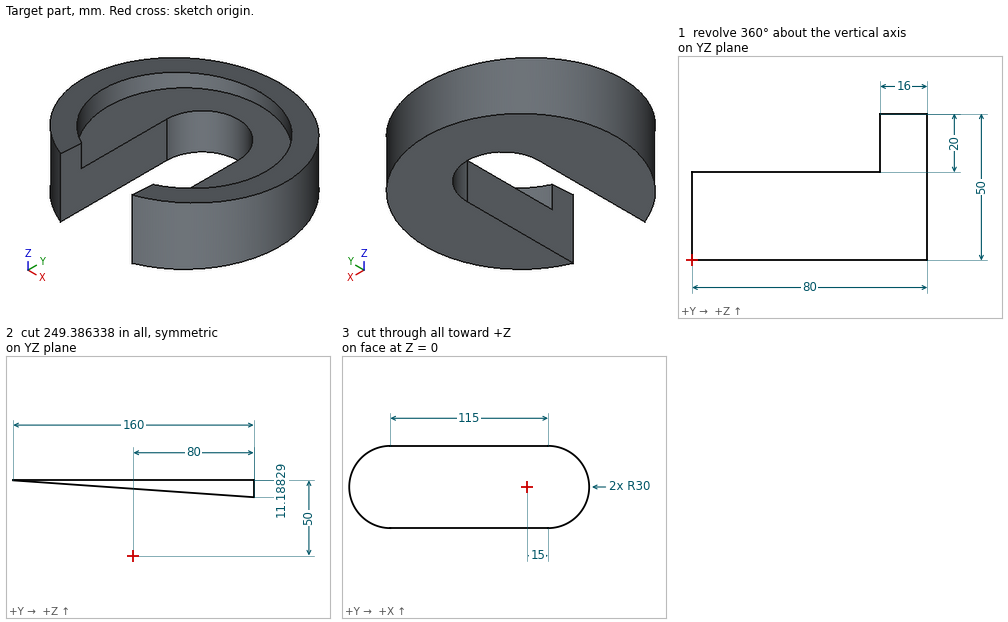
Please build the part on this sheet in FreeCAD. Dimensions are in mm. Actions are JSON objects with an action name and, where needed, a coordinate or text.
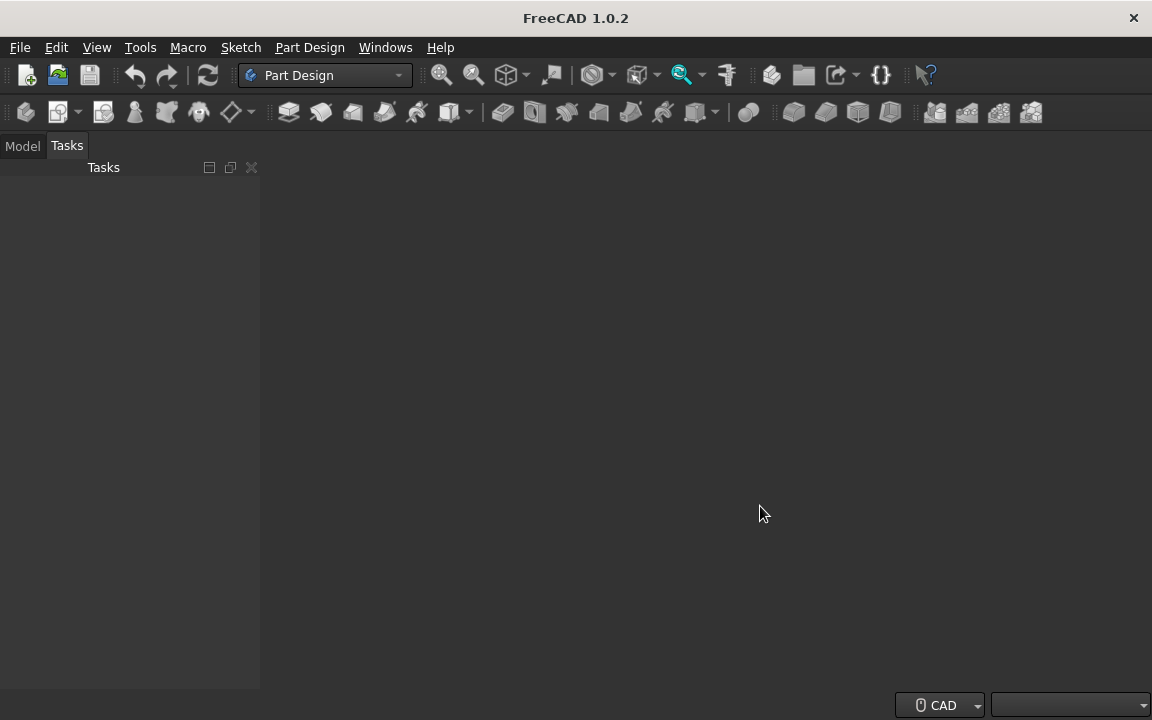
{"action": "left_click", "coordinate": [26, 76]}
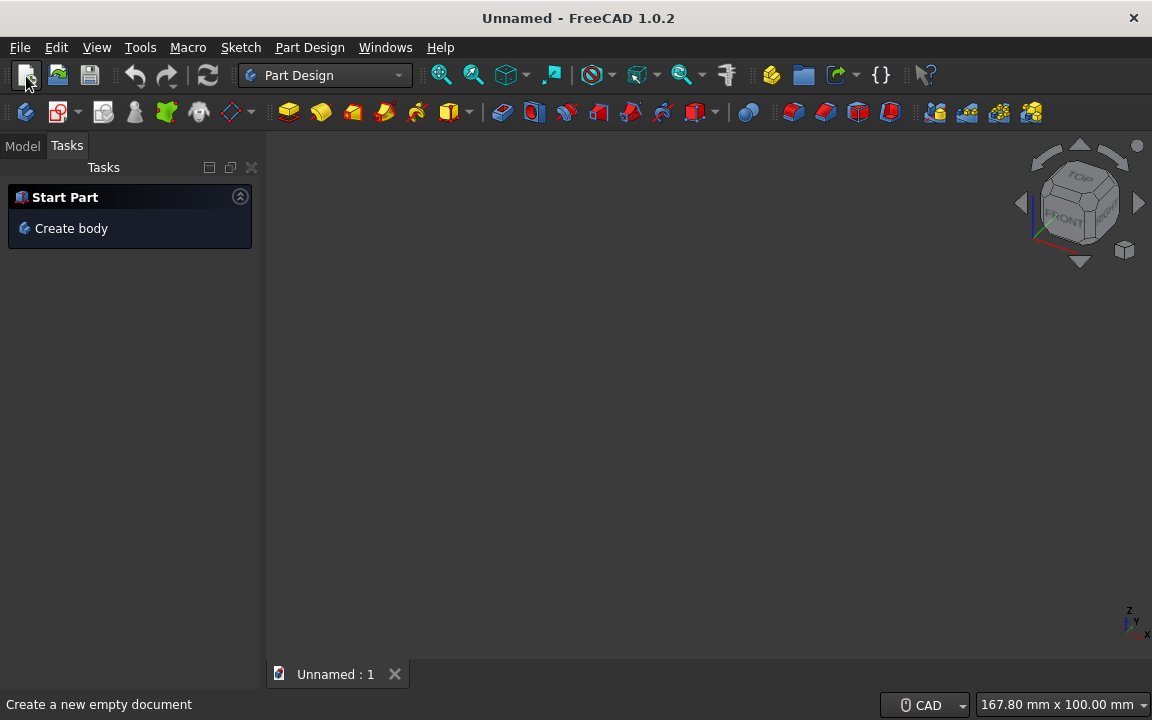
{"action": "left_click", "coordinate": [58, 112]}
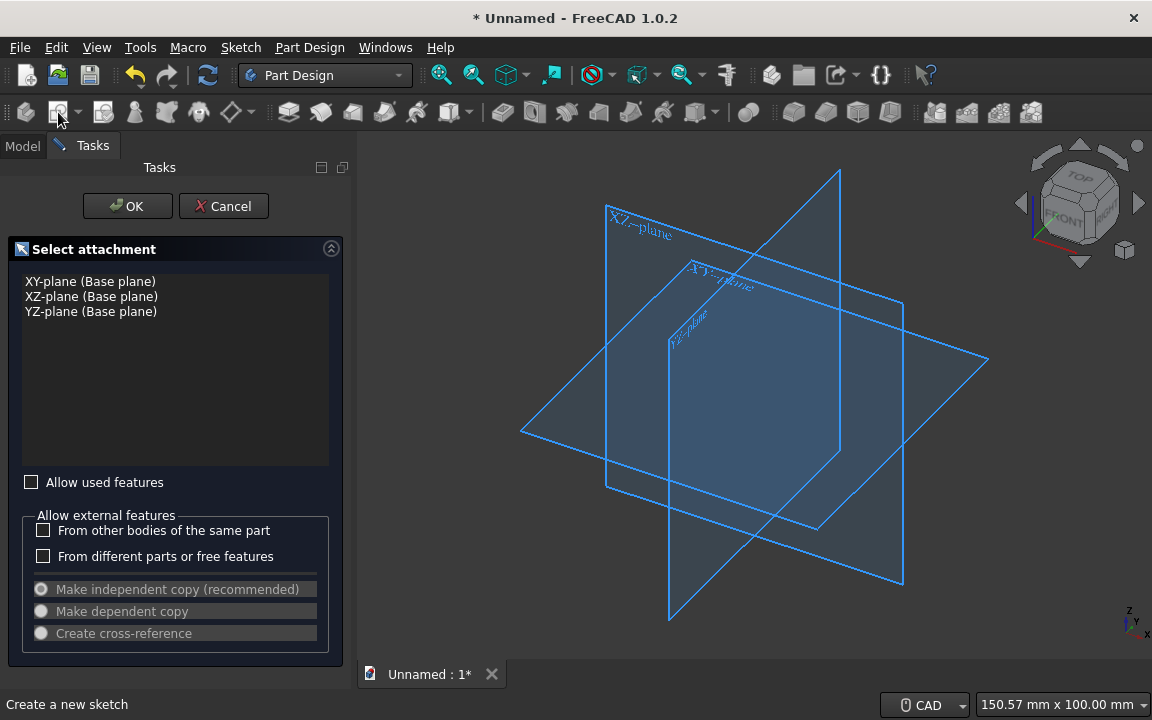
{"action": "left_click", "coordinate": [82, 312]}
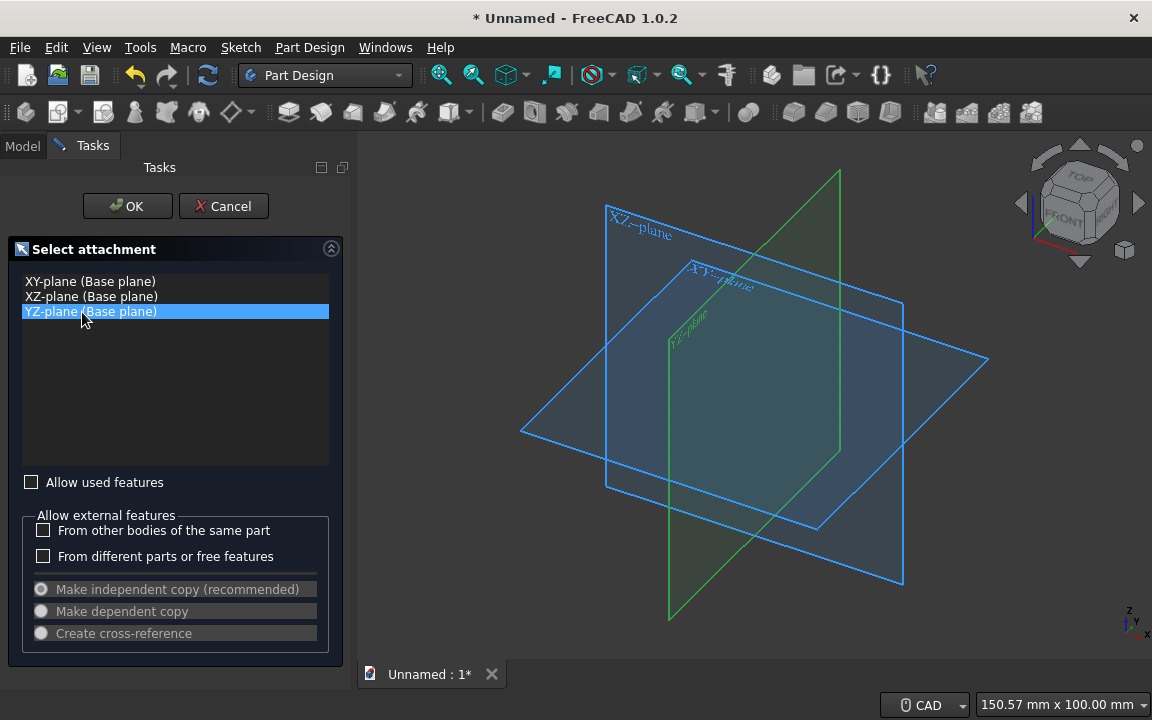
{"action": "left_click", "coordinate": [128, 206]}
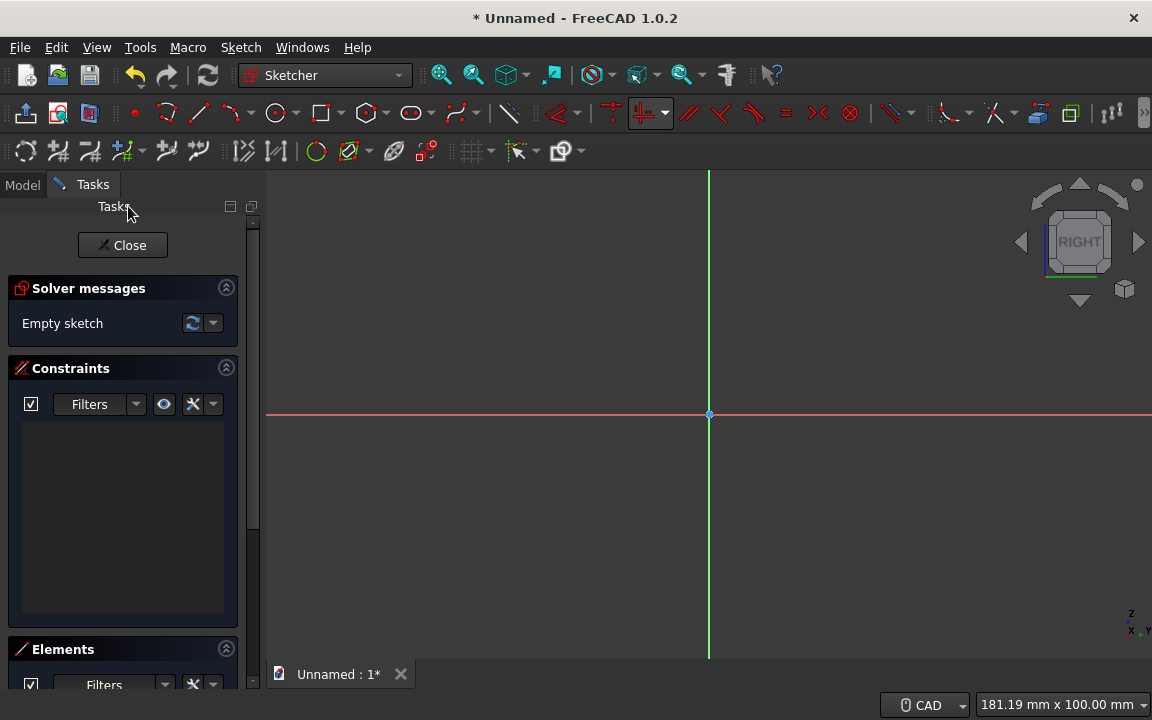
{"action": "scroll", "coordinate": [294, 631], "scroll_direction": "down", "scroll_amount": 1}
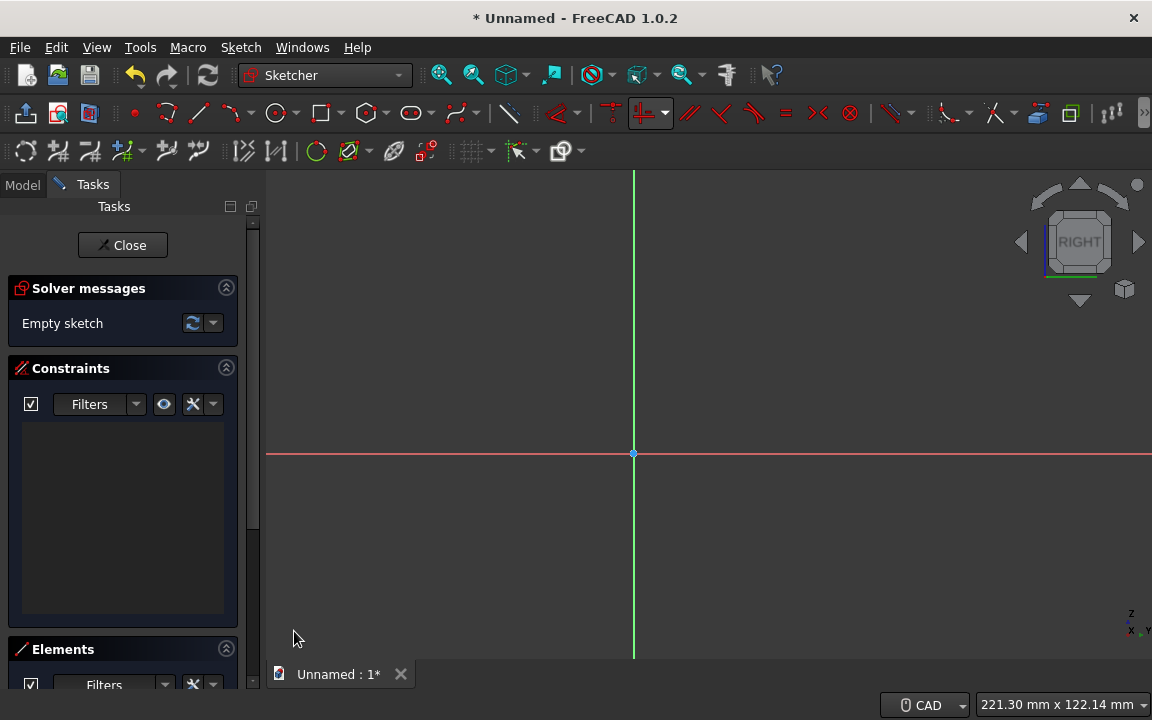
{"action": "scroll", "coordinate": [987, 230], "scroll_direction": "up", "scroll_amount": 2}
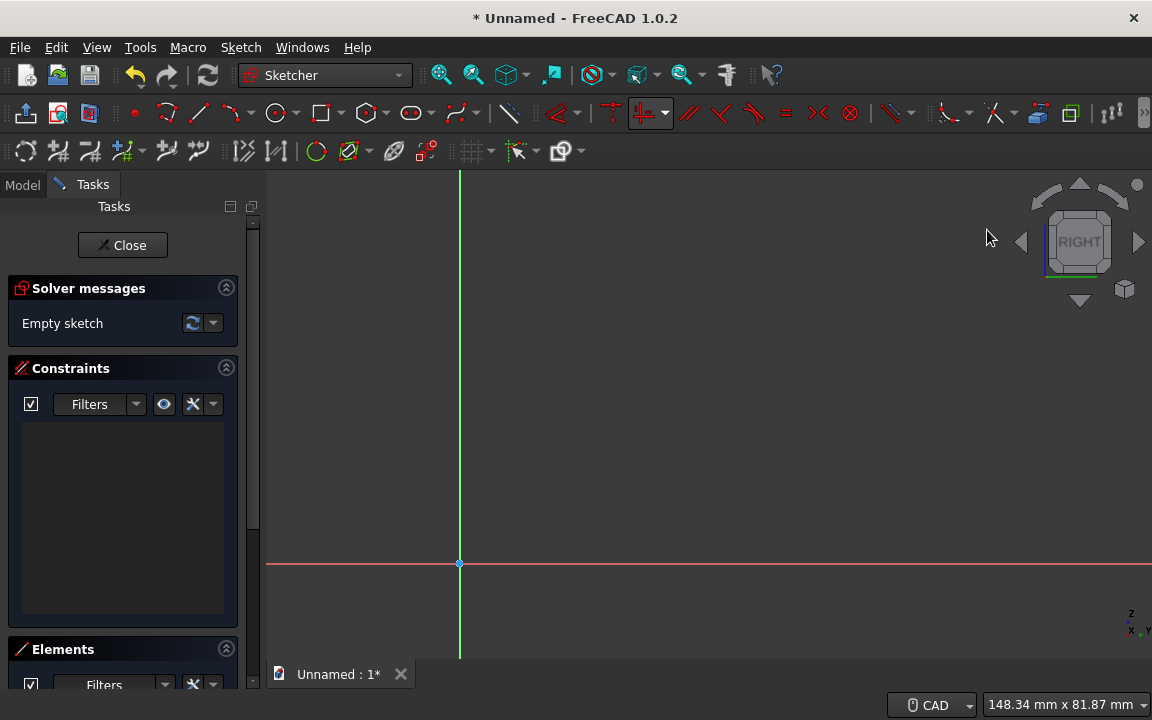
{"action": "left_click", "coordinate": [168, 114]}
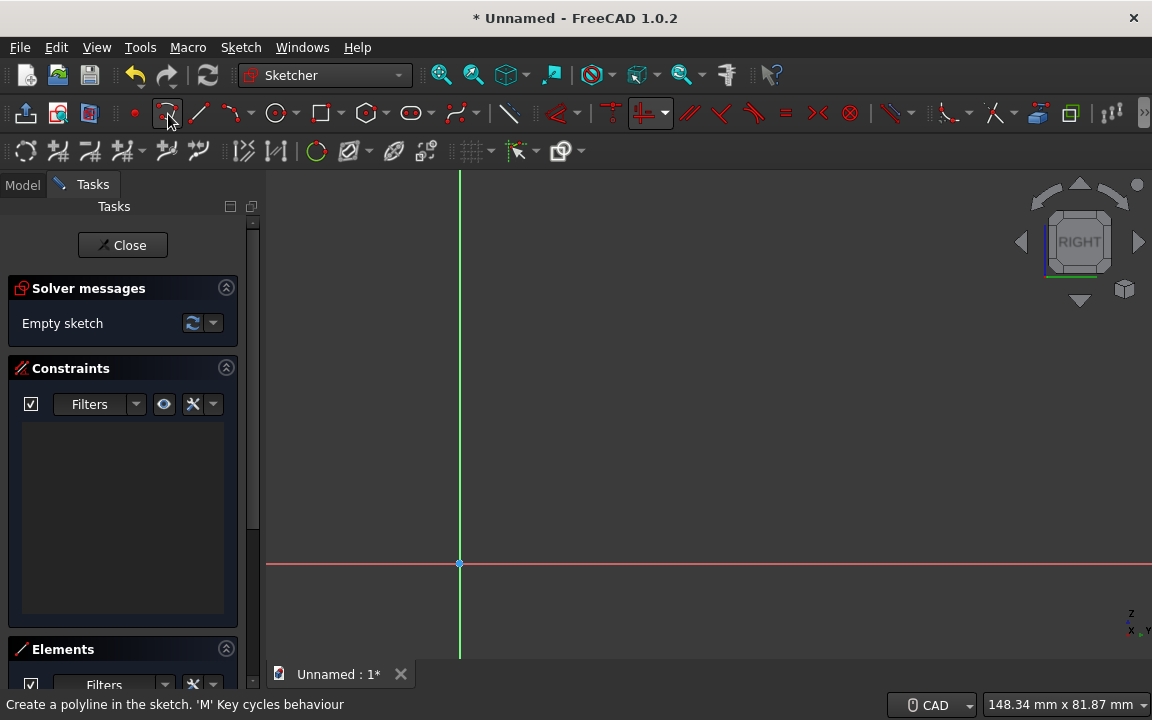
{"action": "left_click", "coordinate": [460, 564]}
{"action": "left_click", "coordinate": [937, 555]}
{"action": "left_click", "coordinate": [937, 265]}
{"action": "left_click", "coordinate": [842, 265]}
{"action": "left_click", "coordinate": [842, 385]}
{"action": "left_click", "coordinate": [469, 385]}
{"action": "left_click", "coordinate": [460, 564]}
{"action": "key", "text": "Escape"}
{"action": "key", "text": "Escape"}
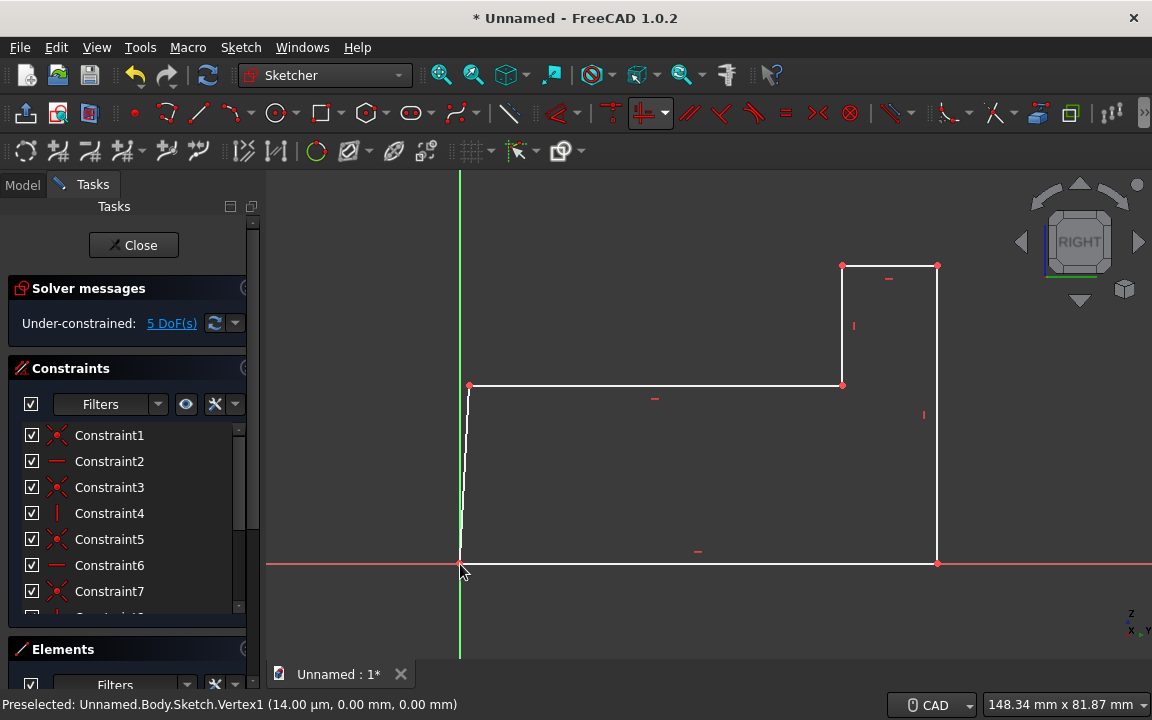
{"action": "left_click", "coordinate": [462, 511]}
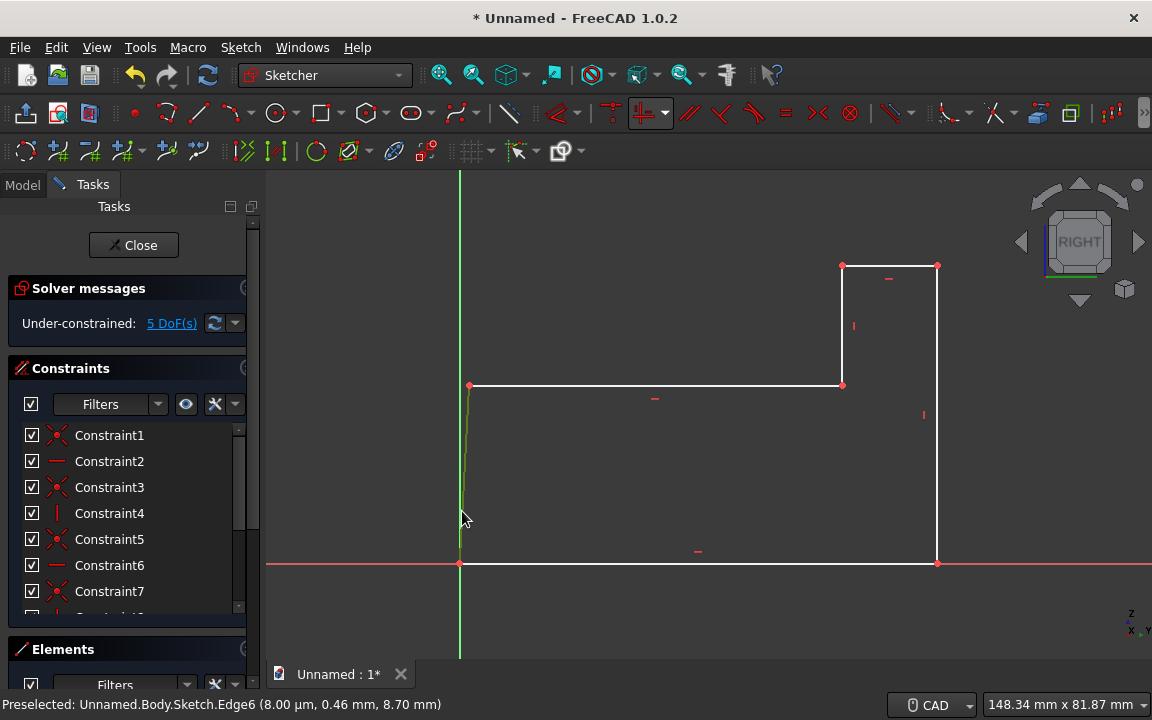
{"action": "key", "text": "v"}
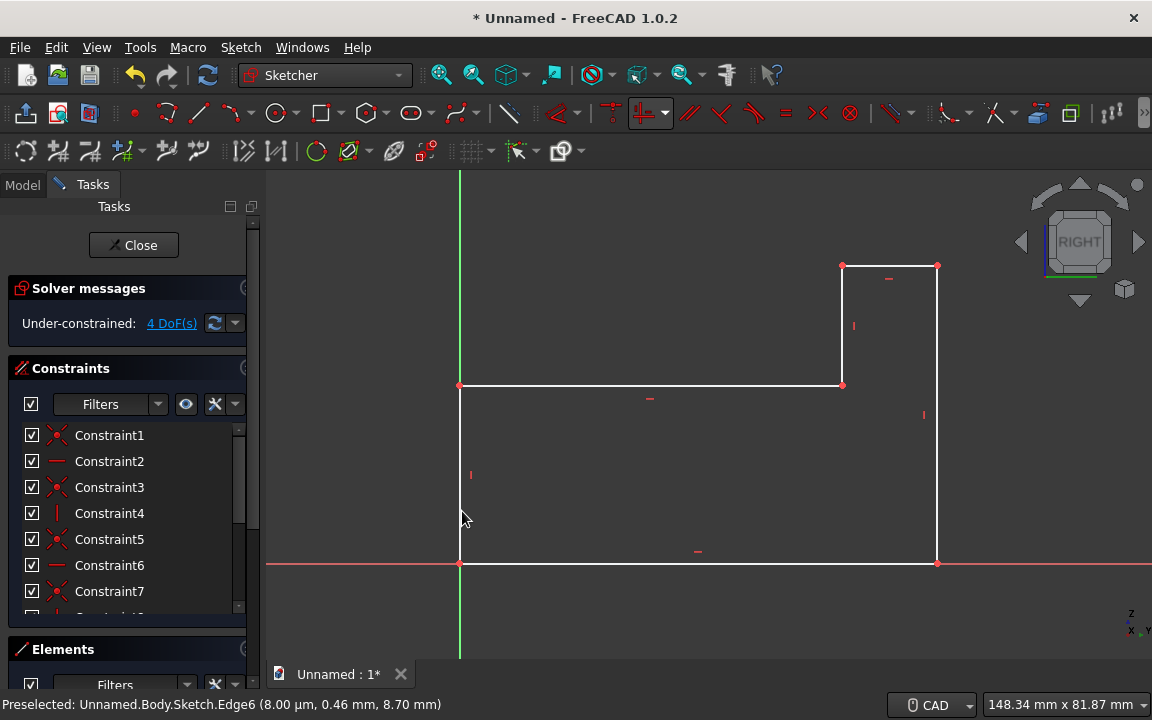
{"action": "left_click", "coordinate": [556, 114]}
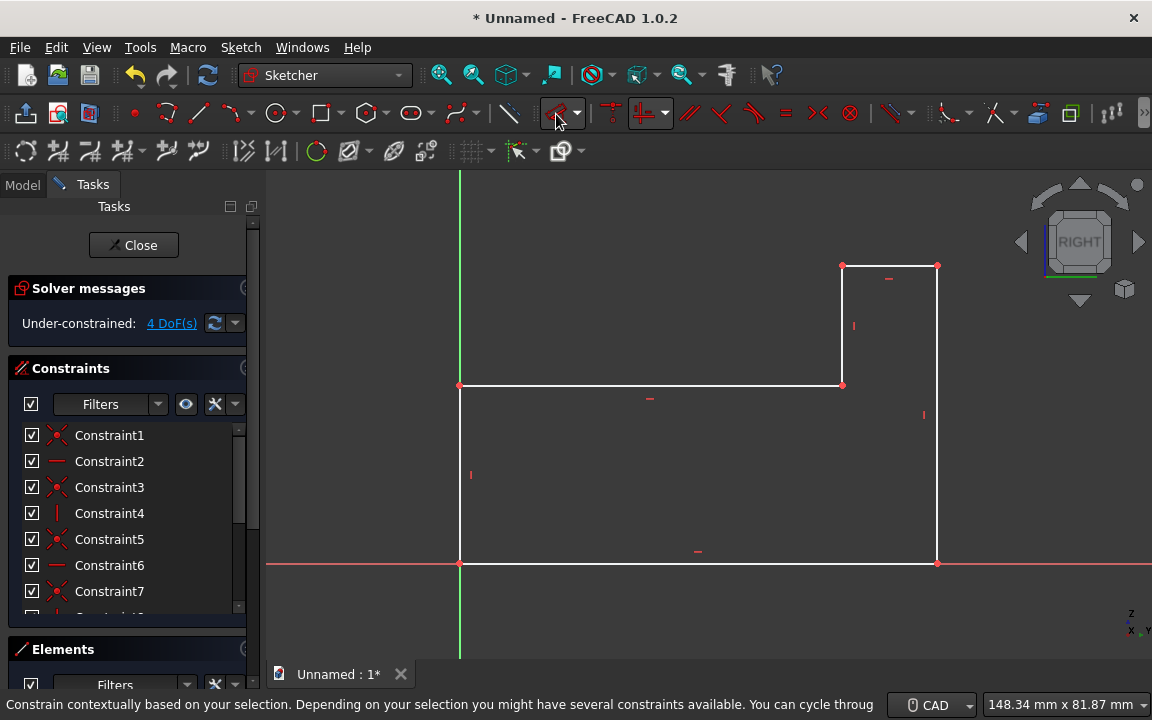
{"action": "left_click", "coordinate": [603, 564]}
{"action": "left_click", "coordinate": [698, 598]}